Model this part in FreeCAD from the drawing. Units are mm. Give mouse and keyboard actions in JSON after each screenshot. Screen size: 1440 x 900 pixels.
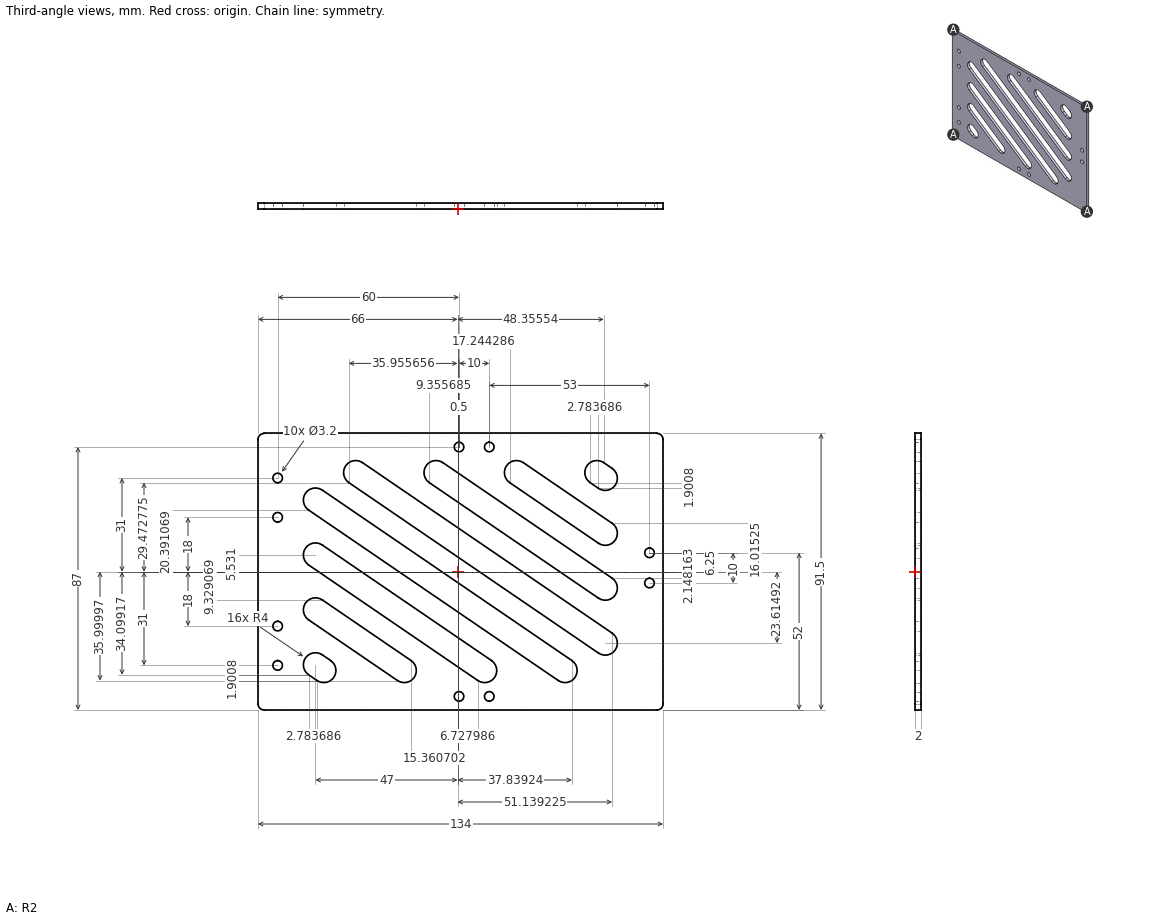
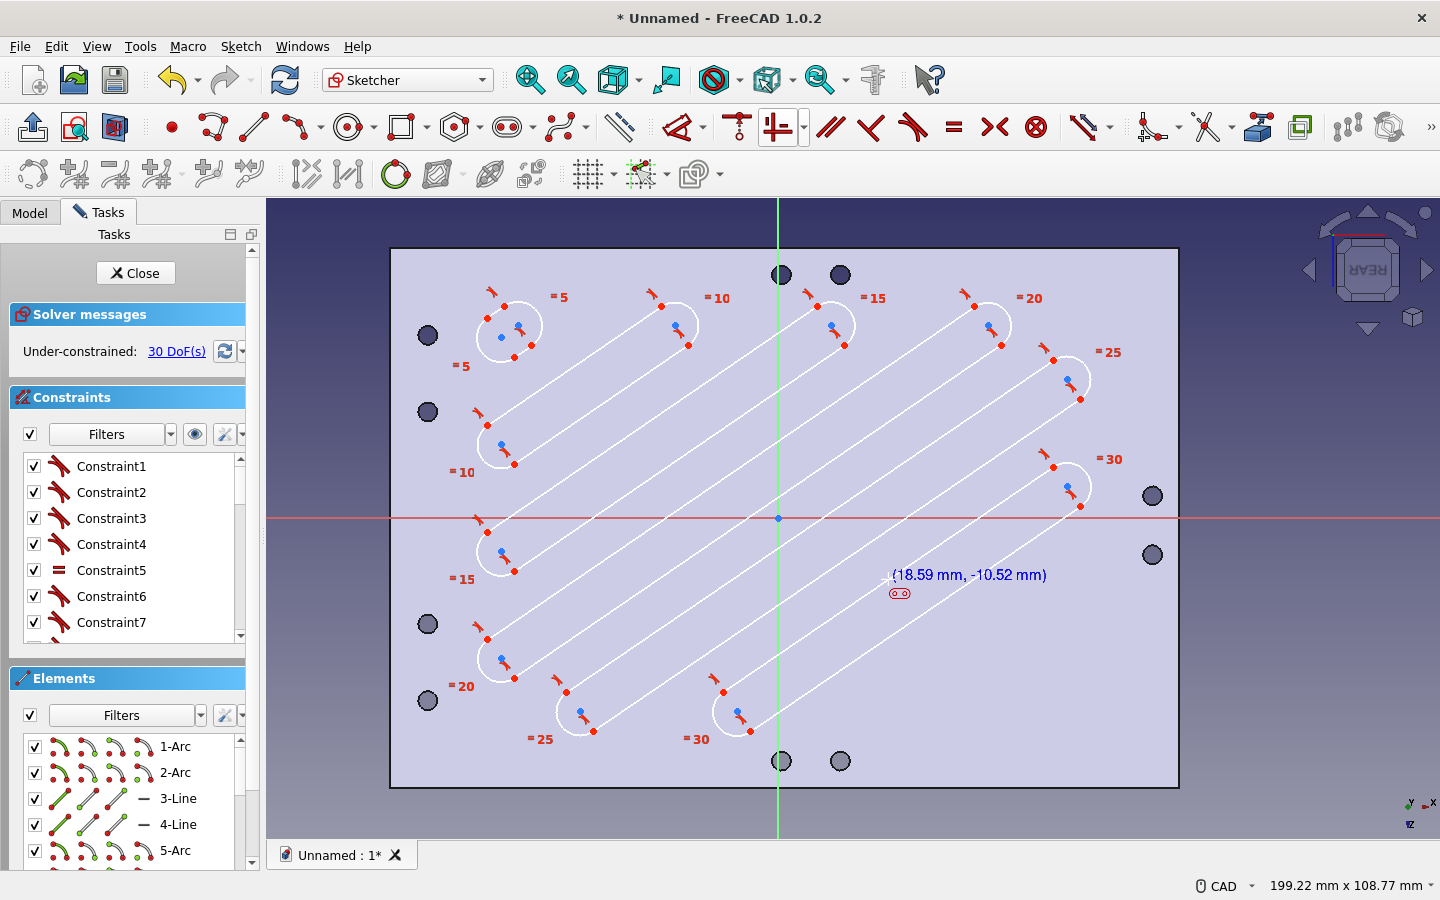
{"action": "left_click", "coordinate": [893, 711]}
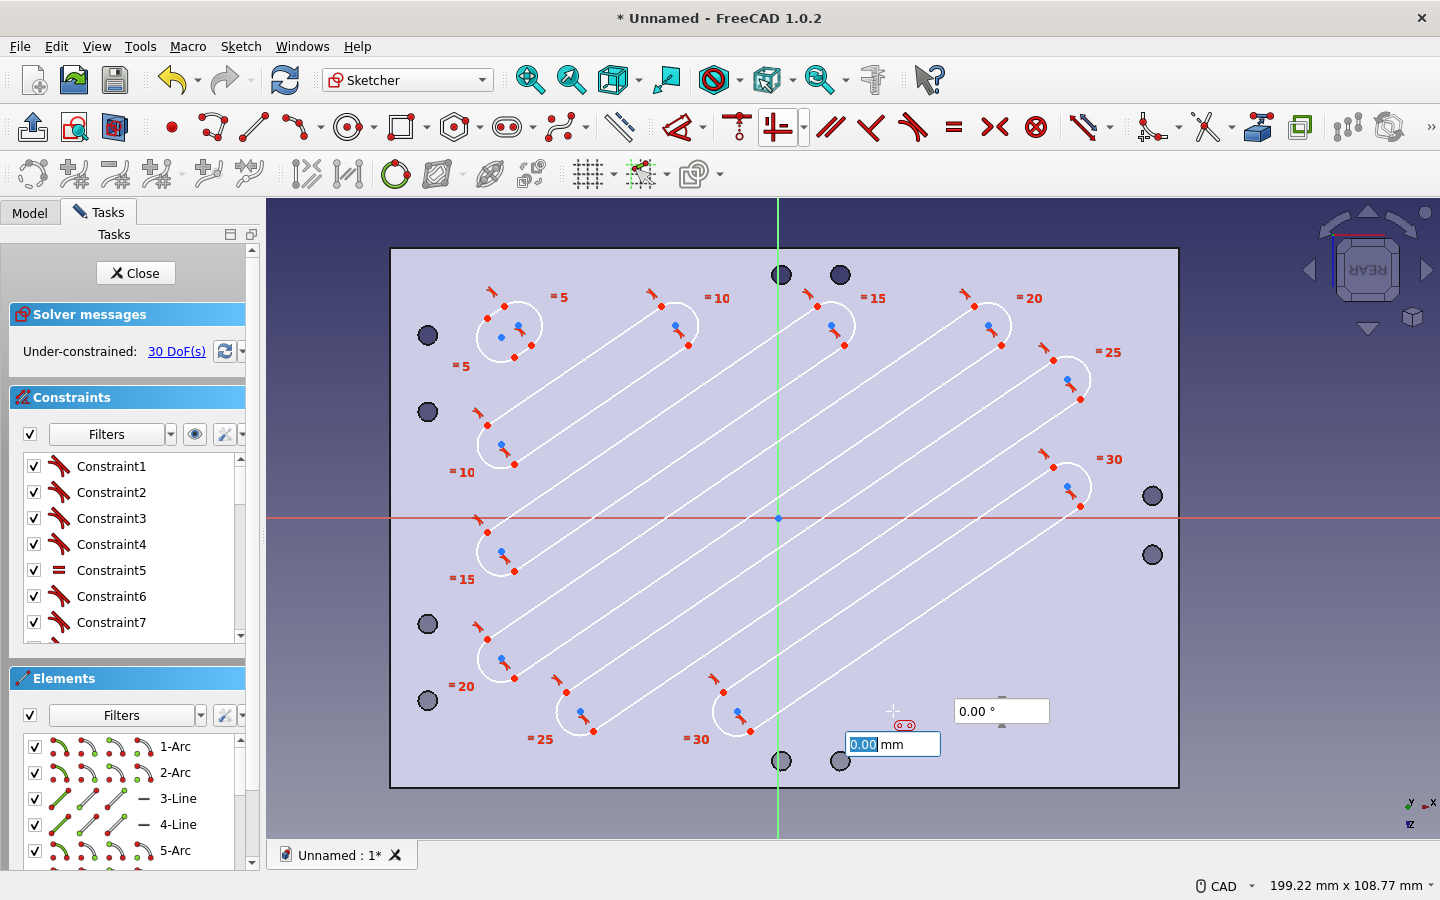
{"action": "left_click", "coordinate": [1067, 593]}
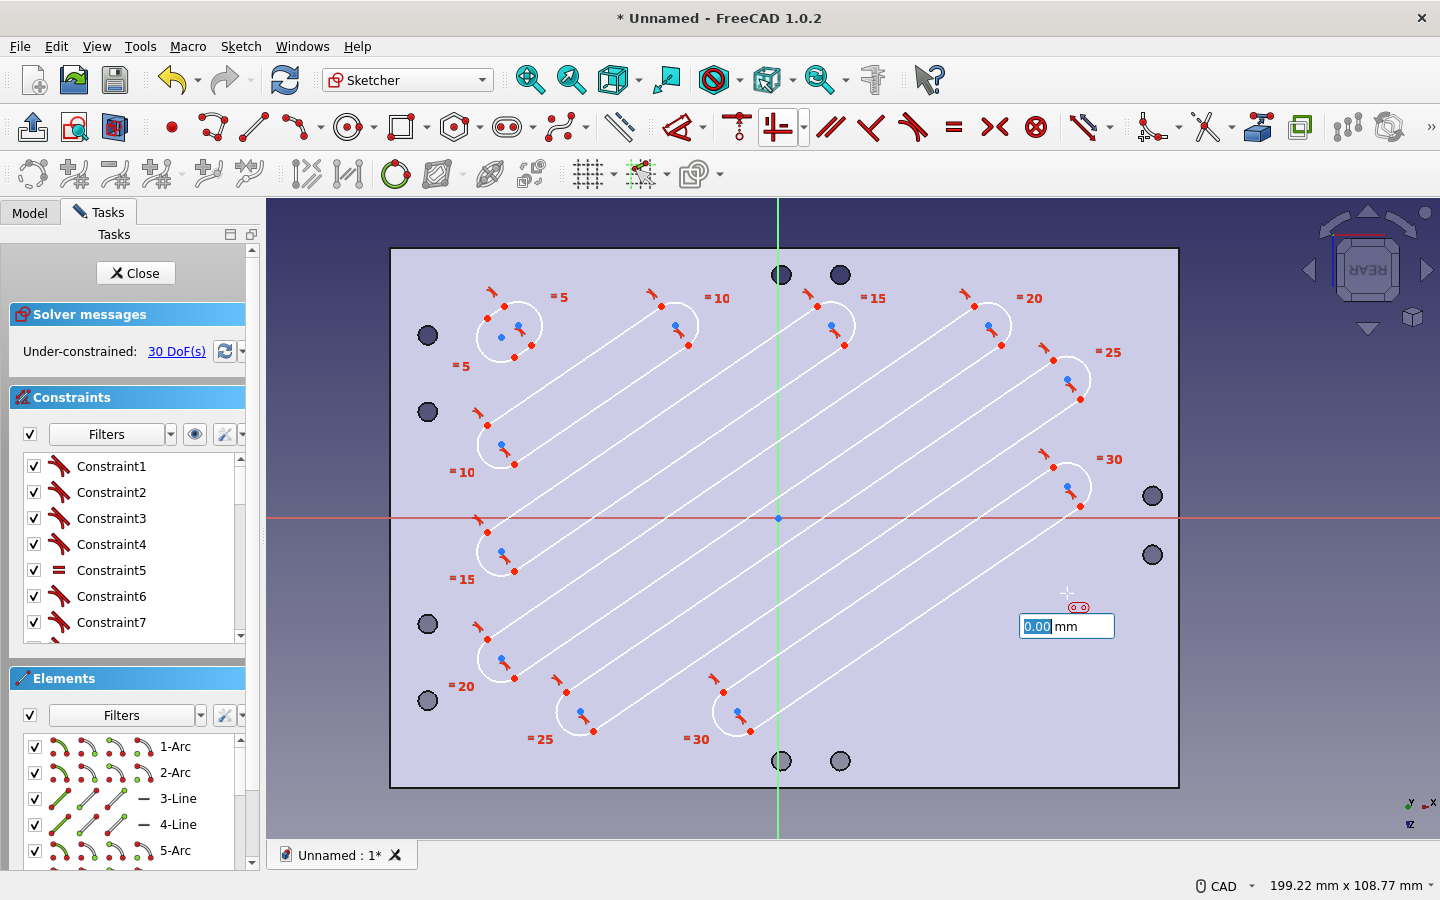
{"action": "left_click", "coordinate": [967, 633]}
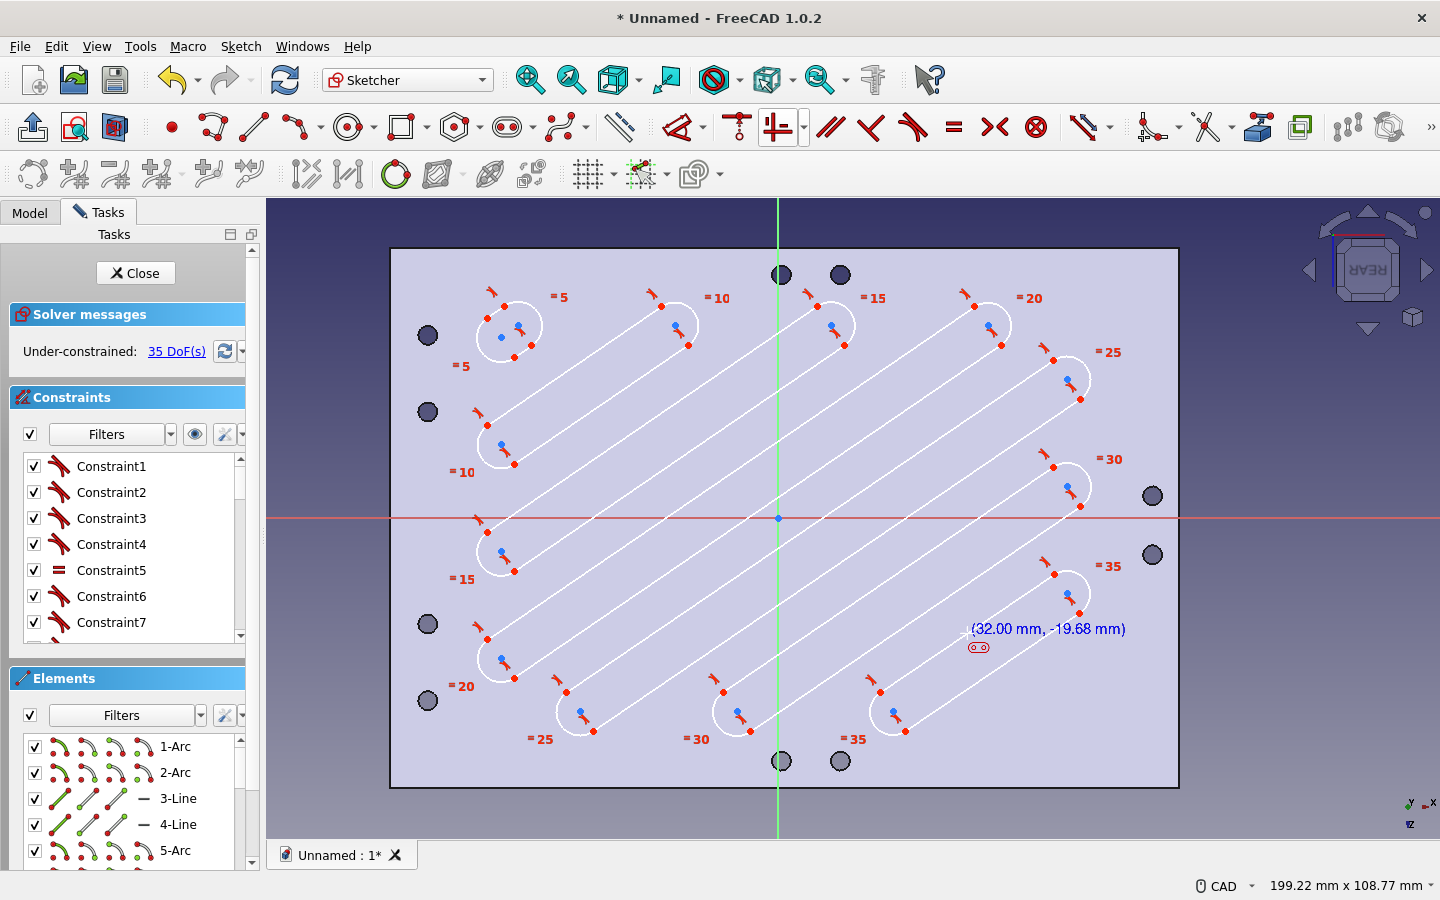
{"action": "left_click", "coordinate": [1050, 711]}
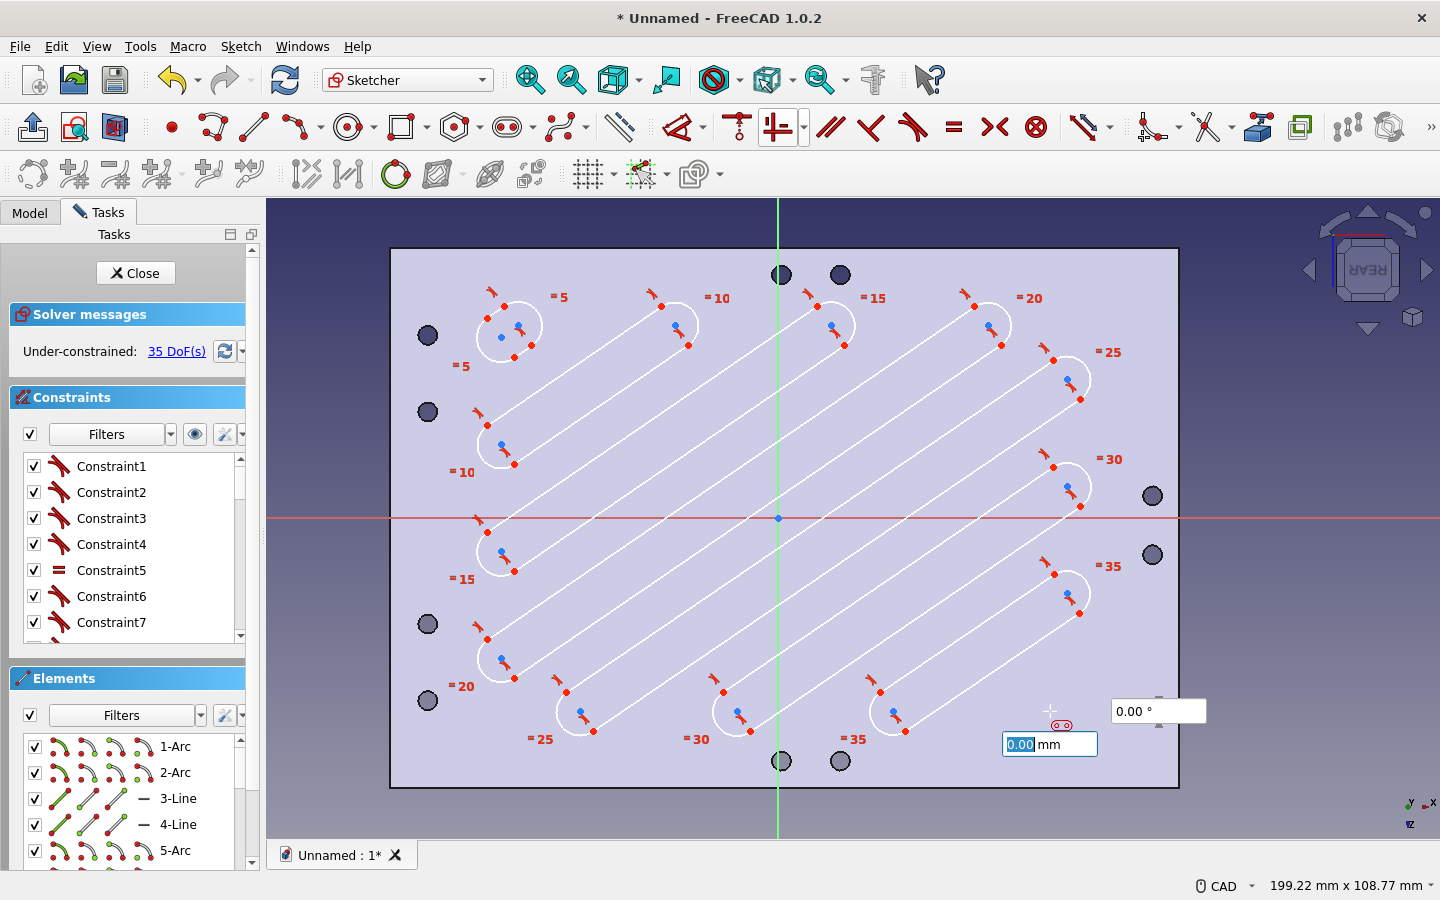
{"action": "left_click", "coordinate": [1067, 700]}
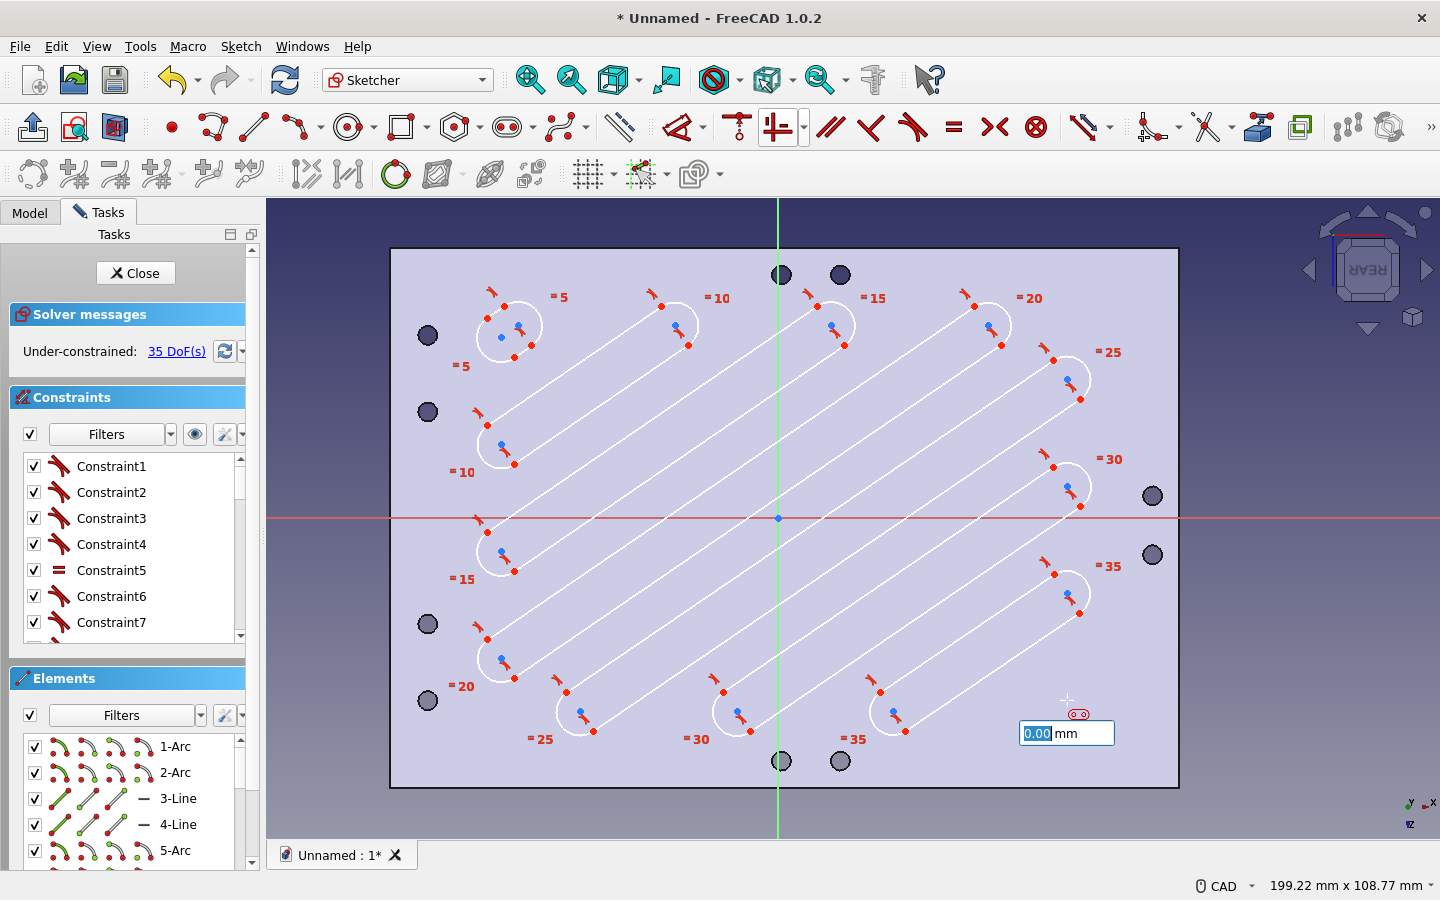
{"action": "left_click", "coordinate": [1045, 686]}
{"action": "key", "text": "Escape"}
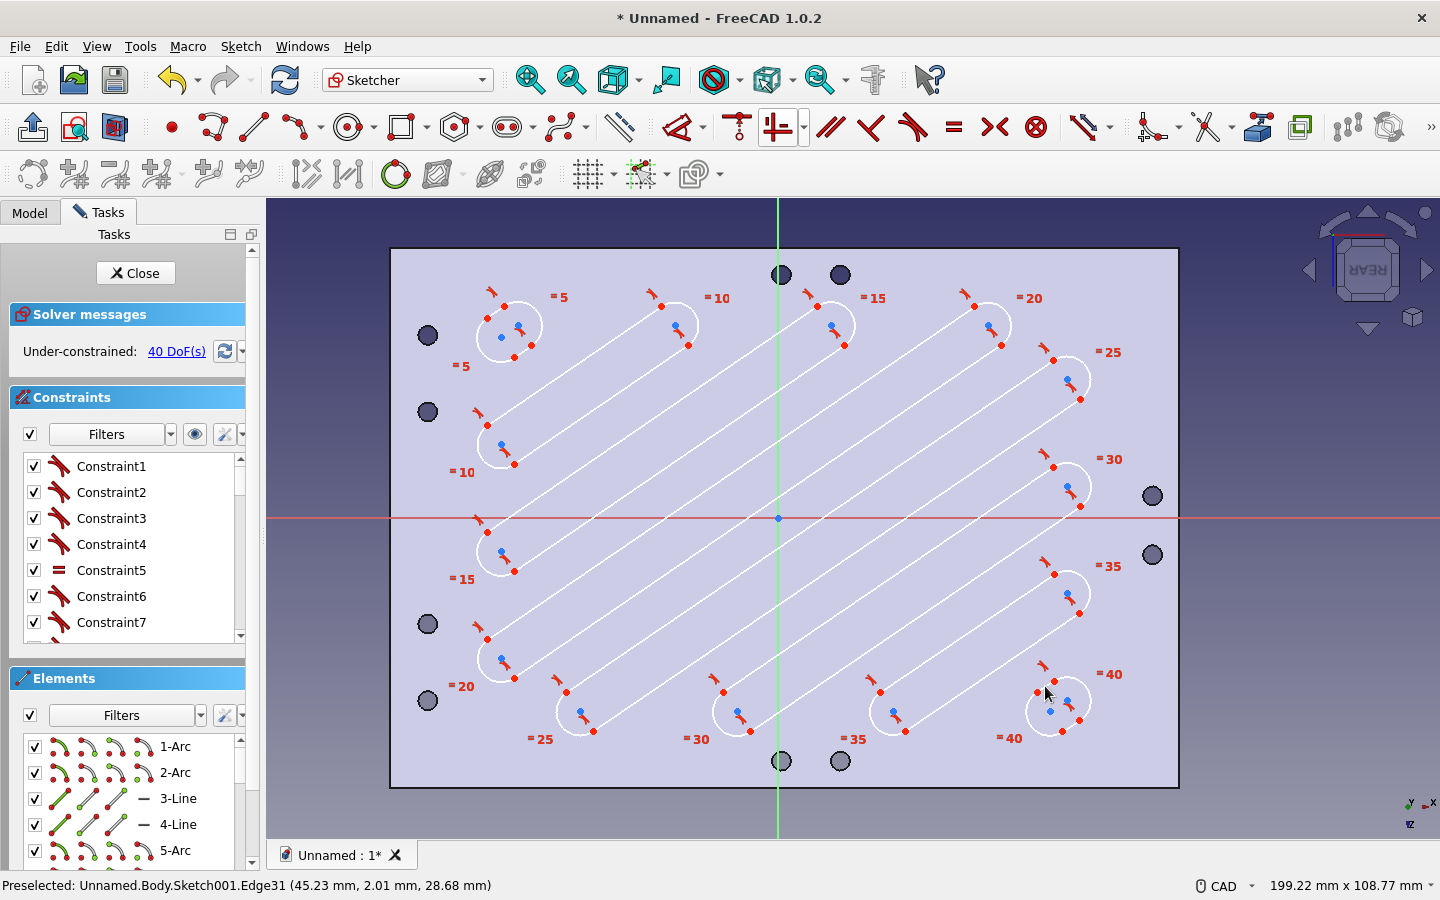
{"action": "left_click", "coordinate": [477, 338]}